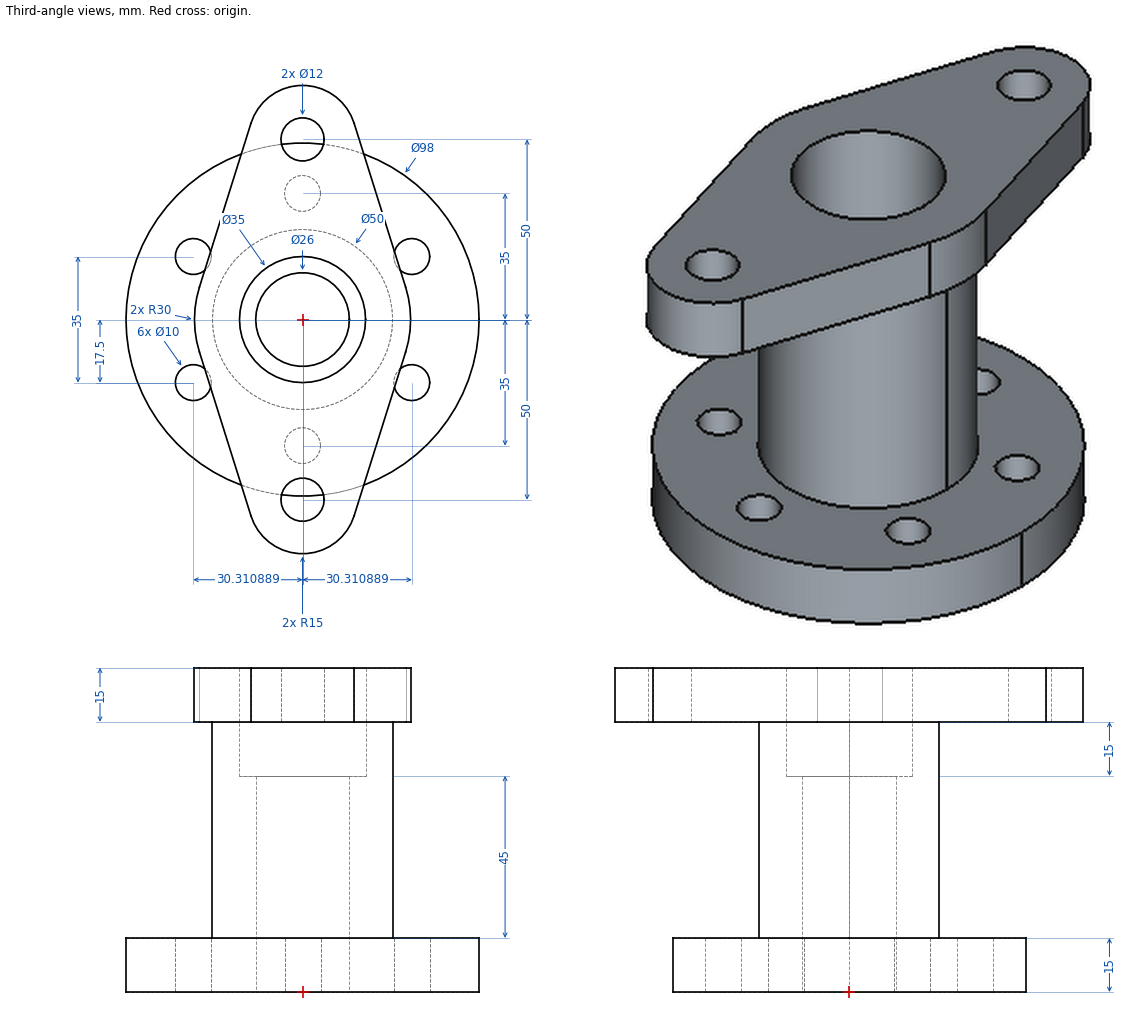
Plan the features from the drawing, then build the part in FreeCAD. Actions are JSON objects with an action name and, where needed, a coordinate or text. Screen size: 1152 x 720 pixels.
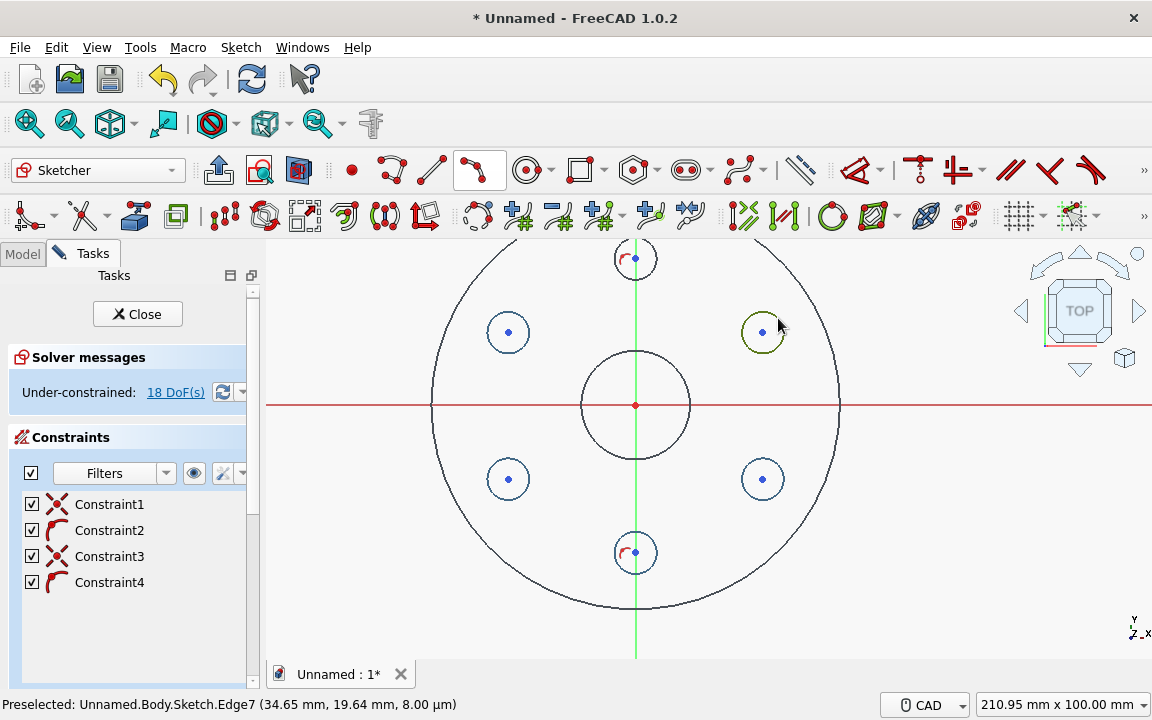
{"action": "left_click", "coordinate": [621, 274]}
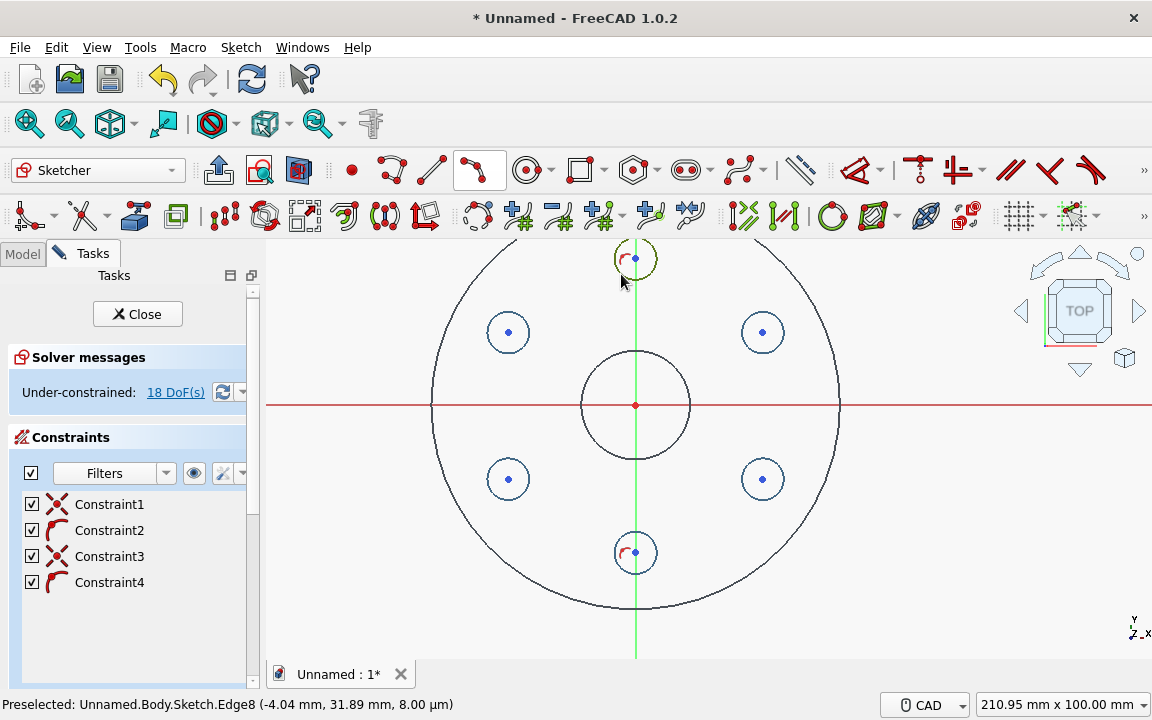
{"action": "key", "text": "e"}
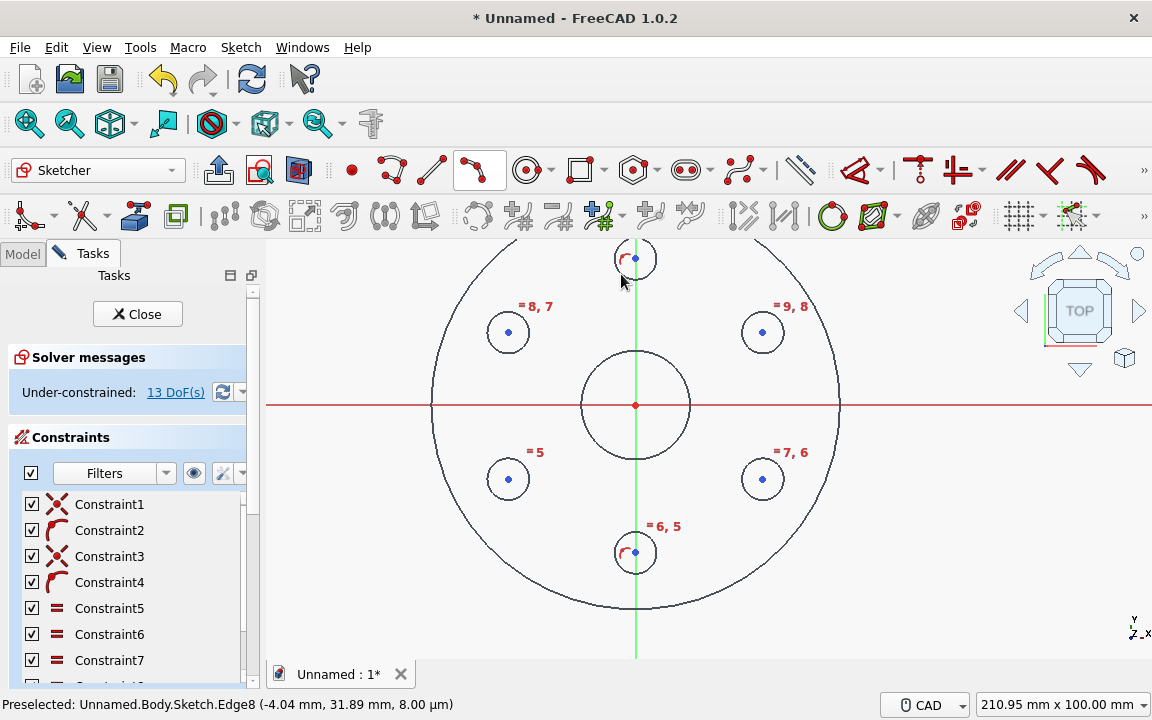
{"action": "left_click", "coordinate": [508, 479]}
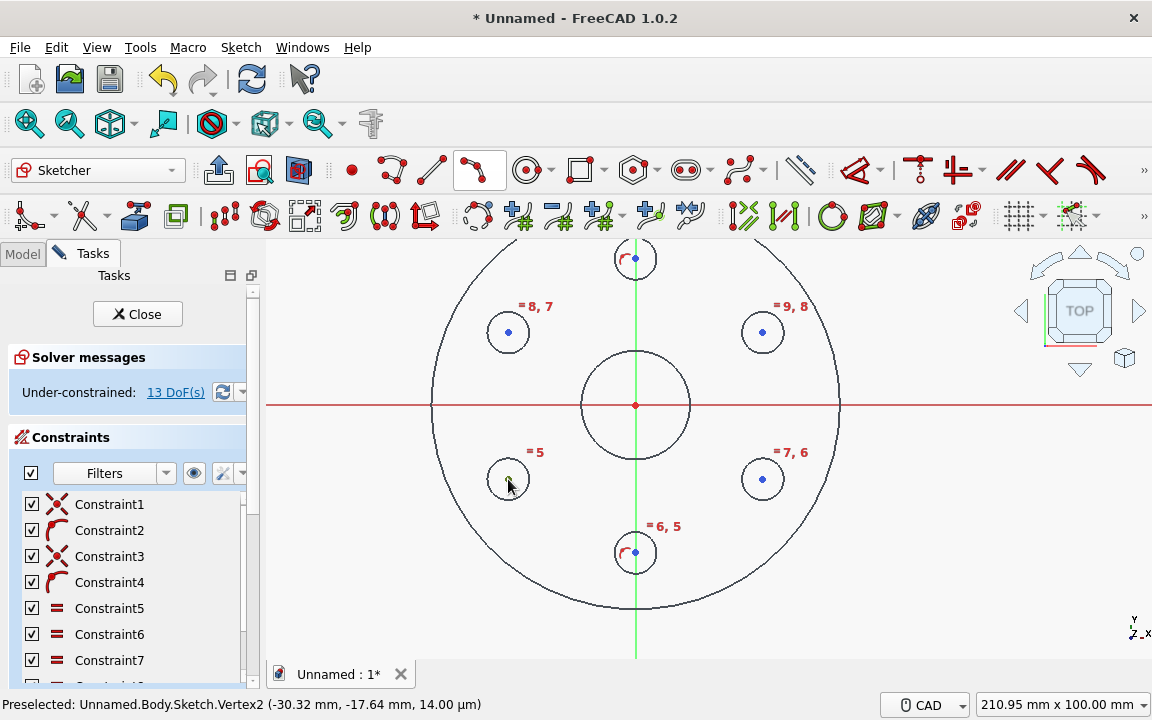
{"action": "left_click", "coordinate": [763, 479]}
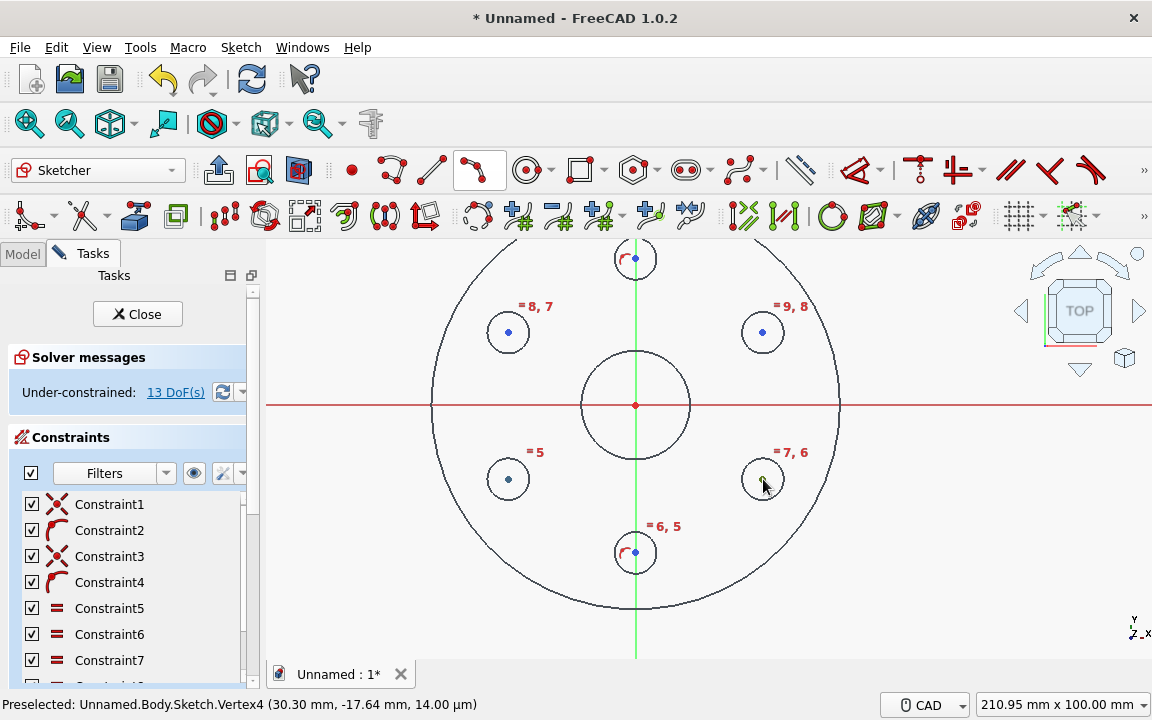
{"action": "key", "text": "h"}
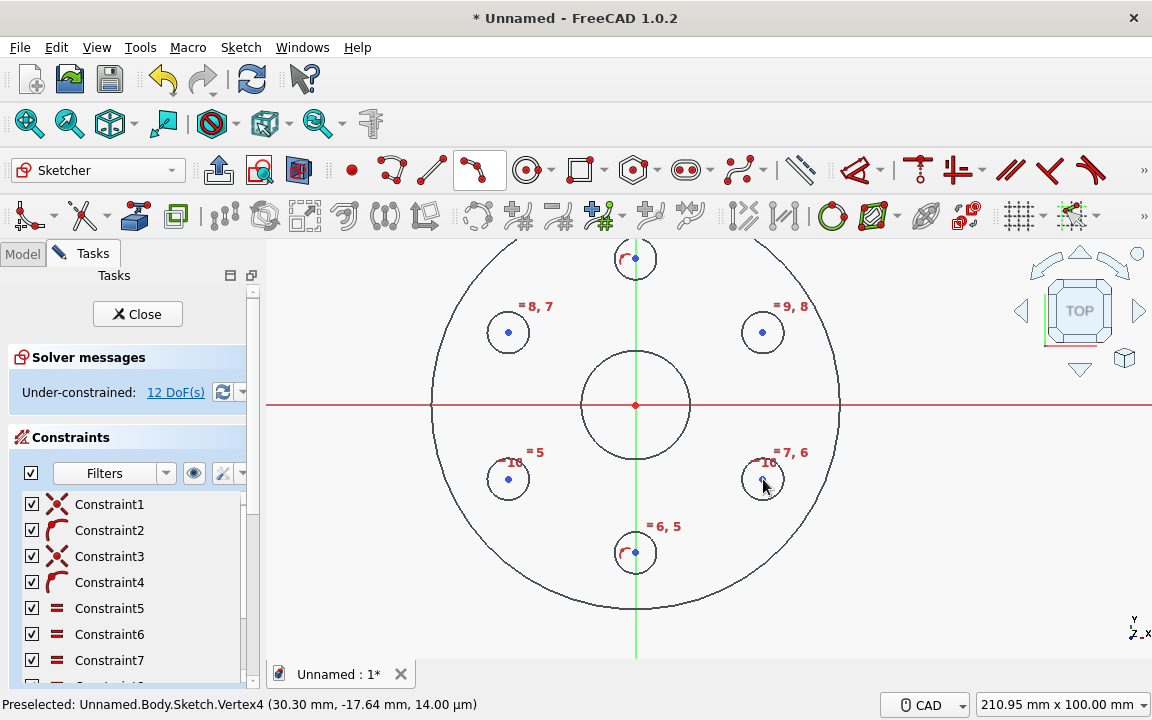
{"action": "left_click", "coordinate": [508, 479]}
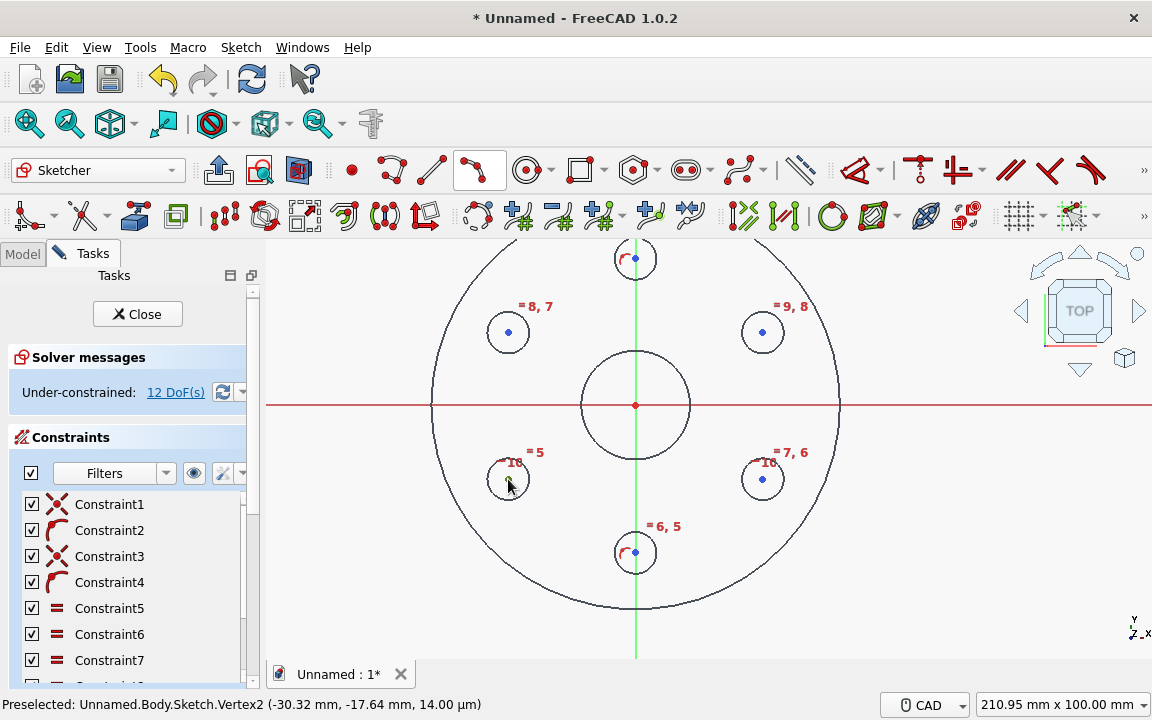
{"action": "left_click", "coordinate": [508, 333]}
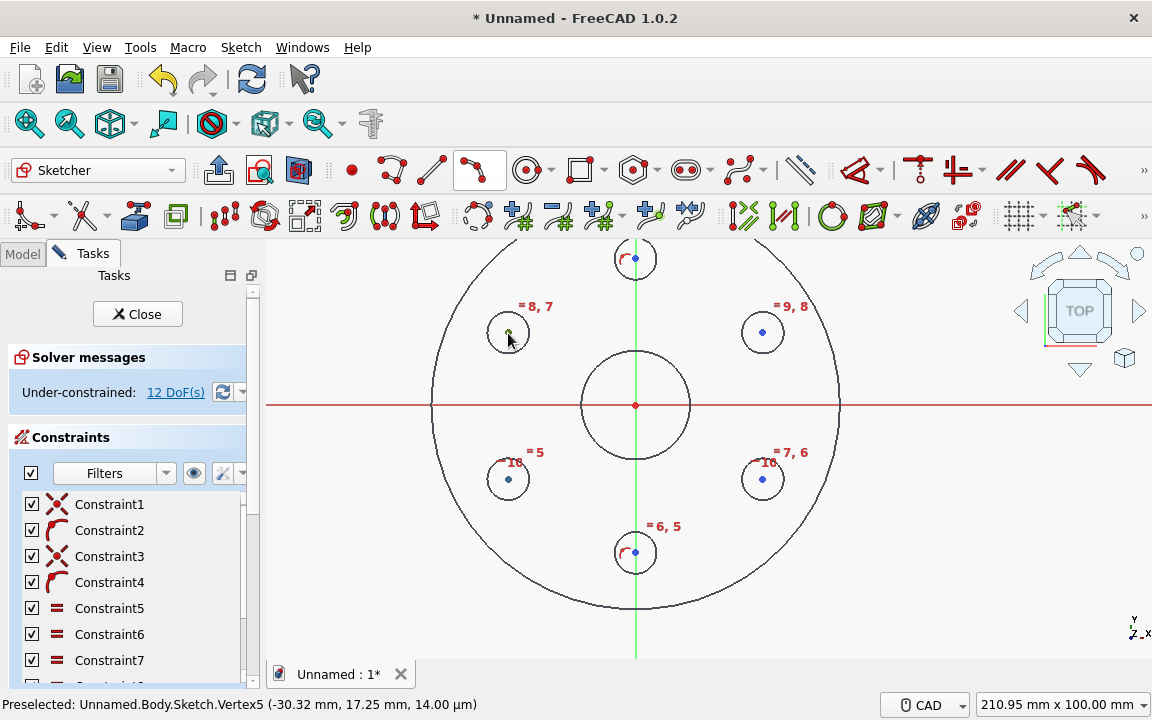
{"action": "key", "text": "v"}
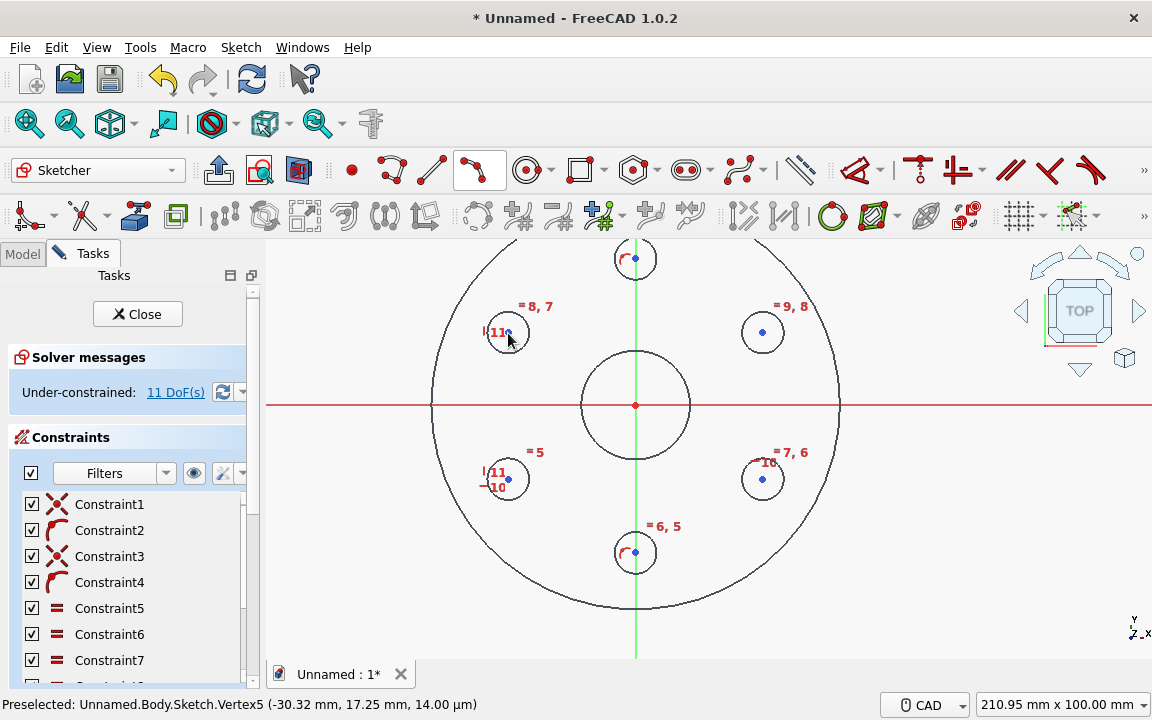
{"action": "left_click", "coordinate": [763, 479]}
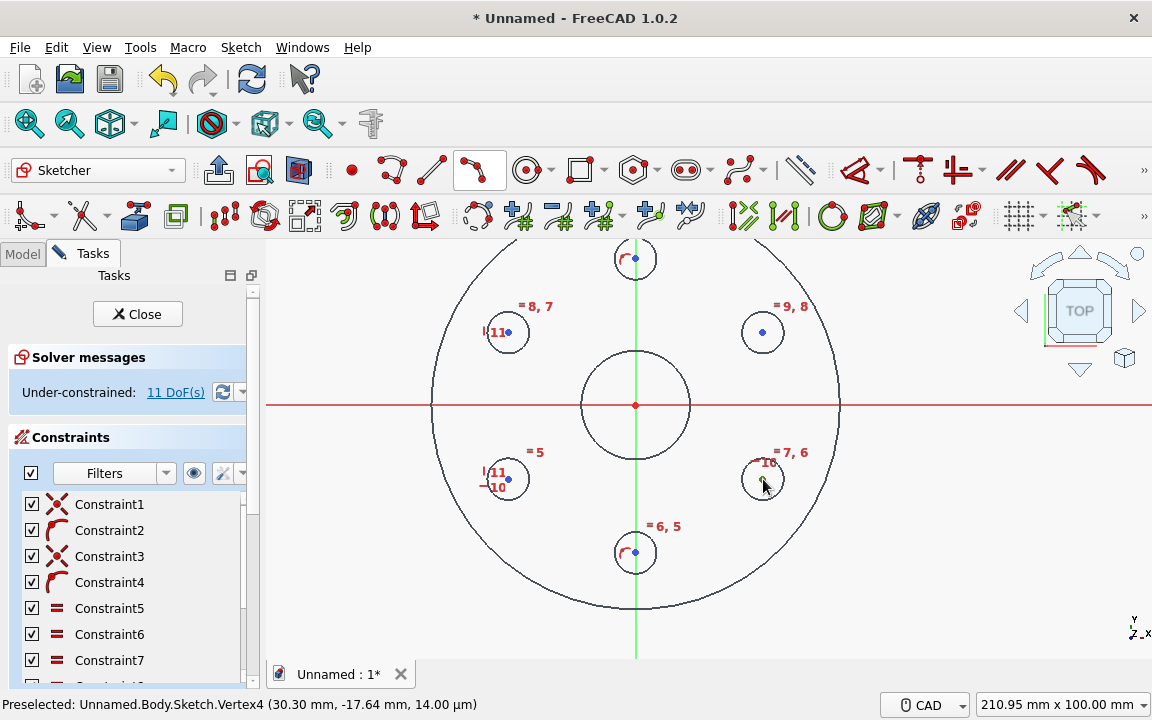
{"action": "left_click", "coordinate": [763, 333]}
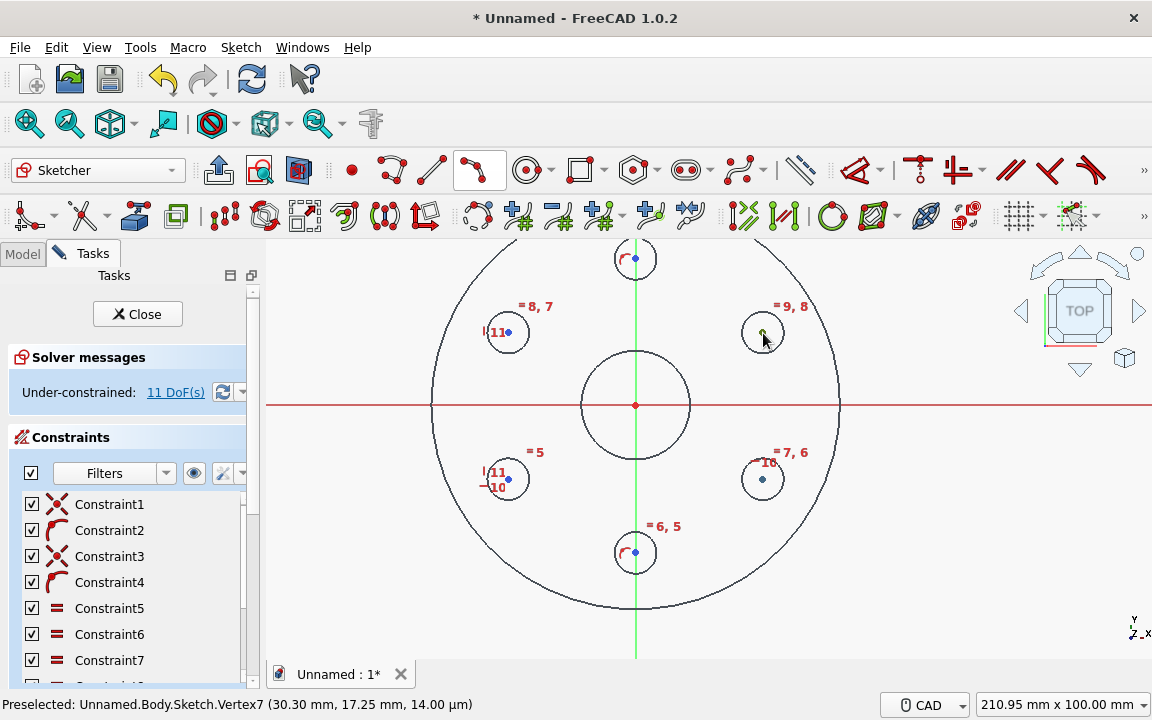
{"action": "key", "text": "v"}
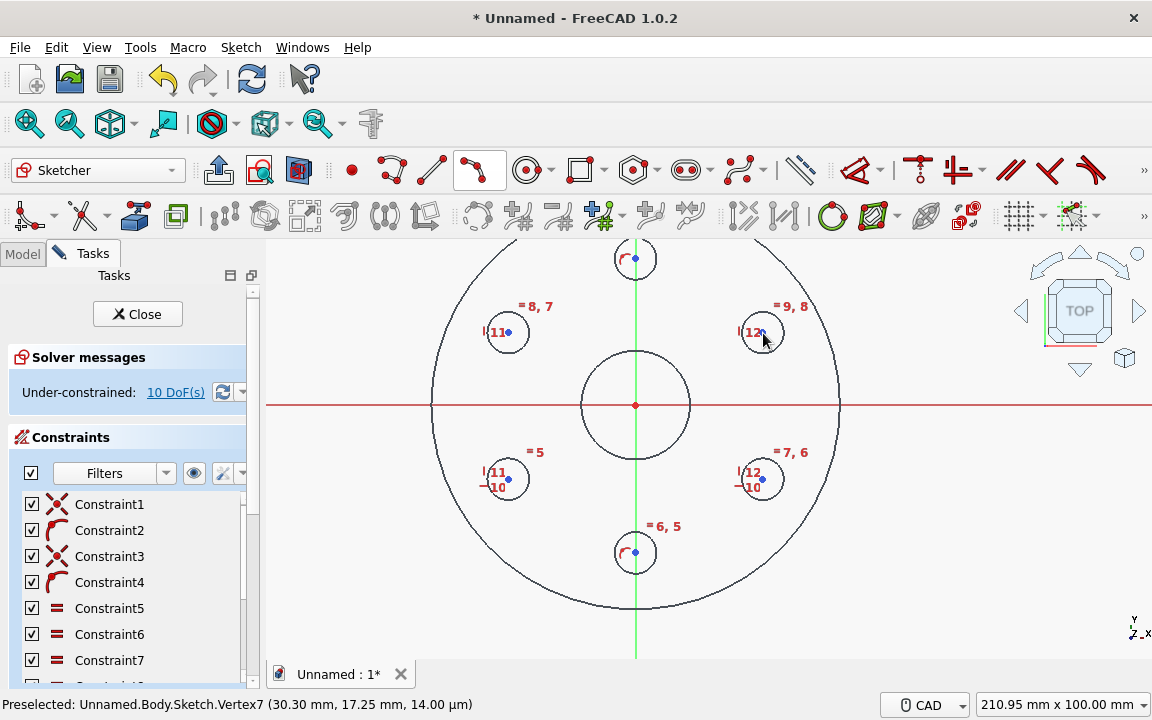
{"action": "left_click", "coordinate": [508, 333]}